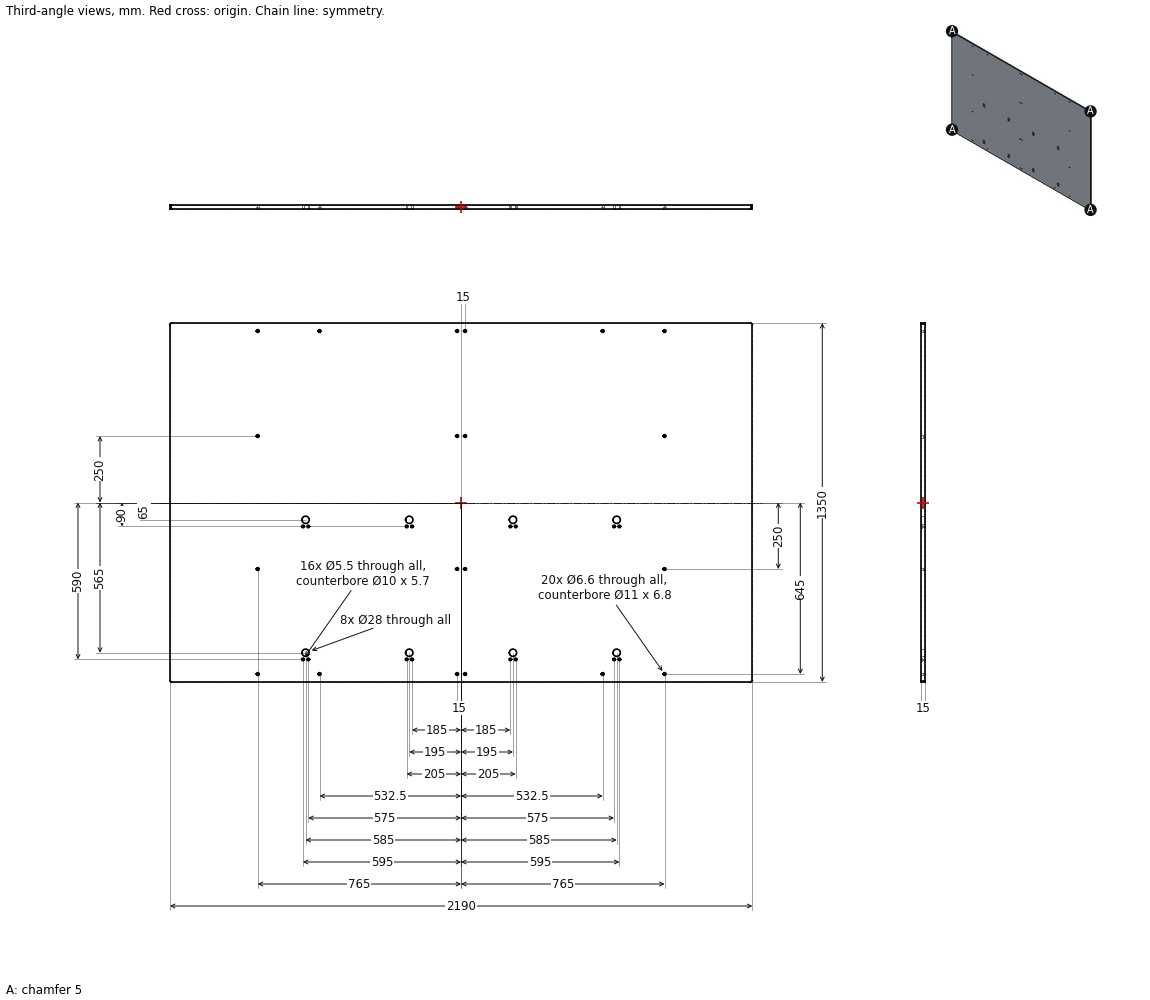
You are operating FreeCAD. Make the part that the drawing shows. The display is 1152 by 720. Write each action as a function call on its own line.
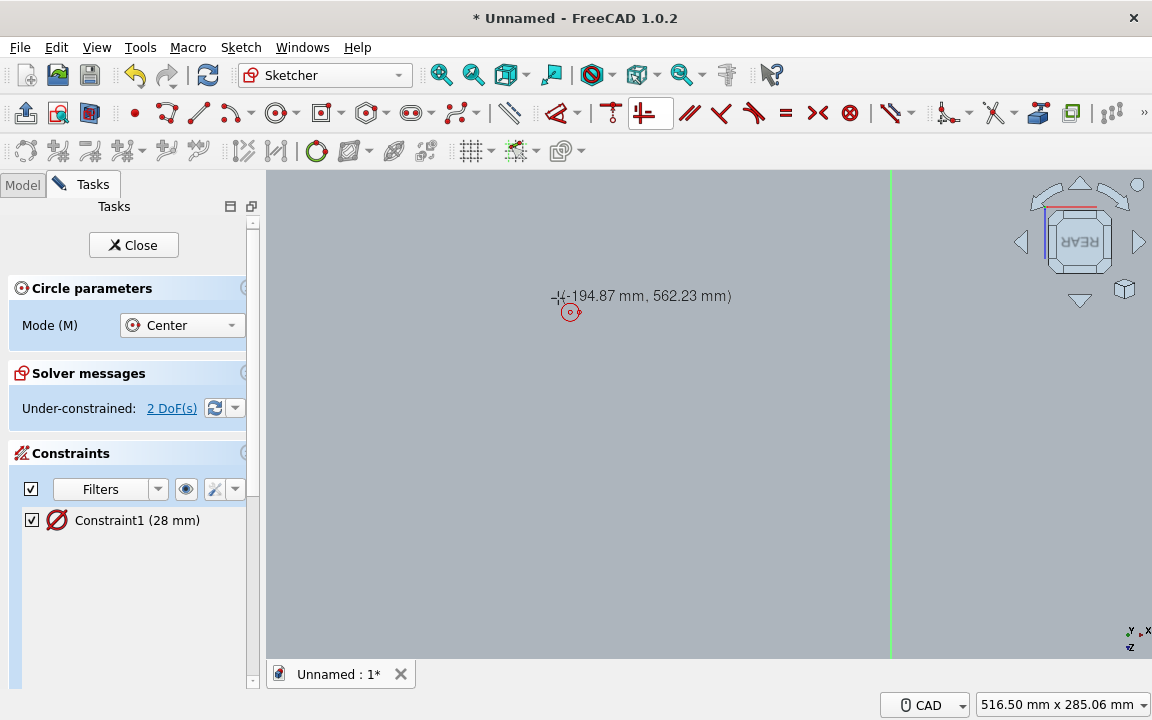
scroll(558, 298, down, 7)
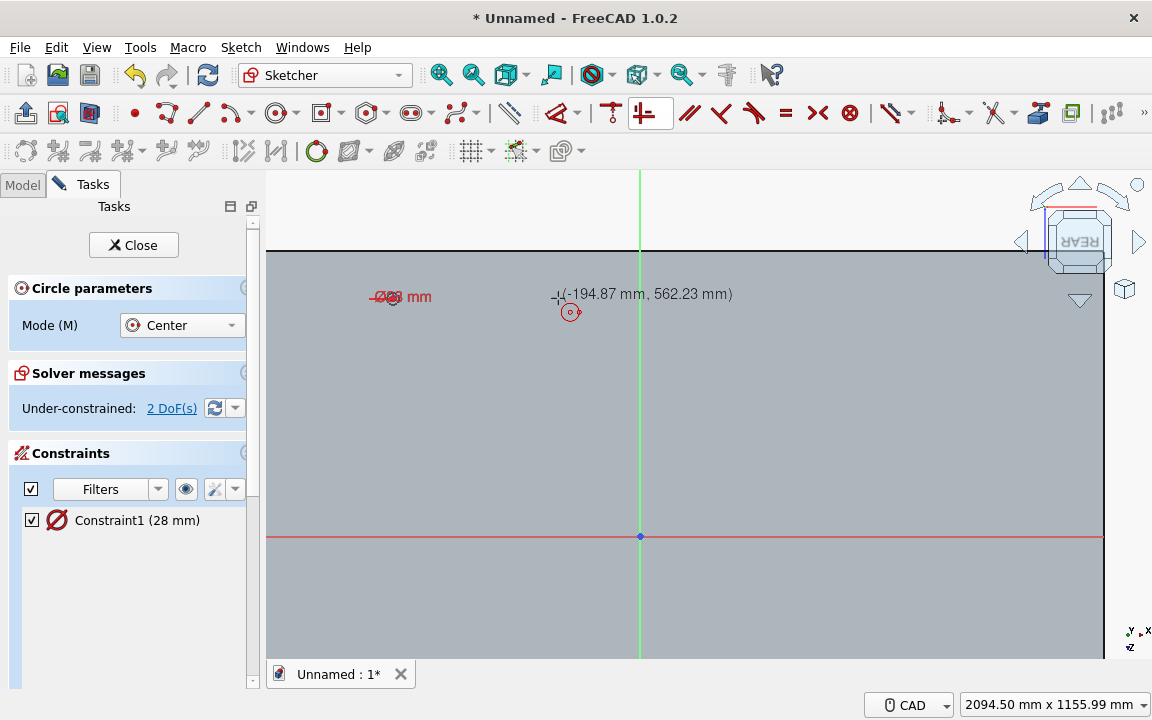
click(558, 298)
move(562, 294)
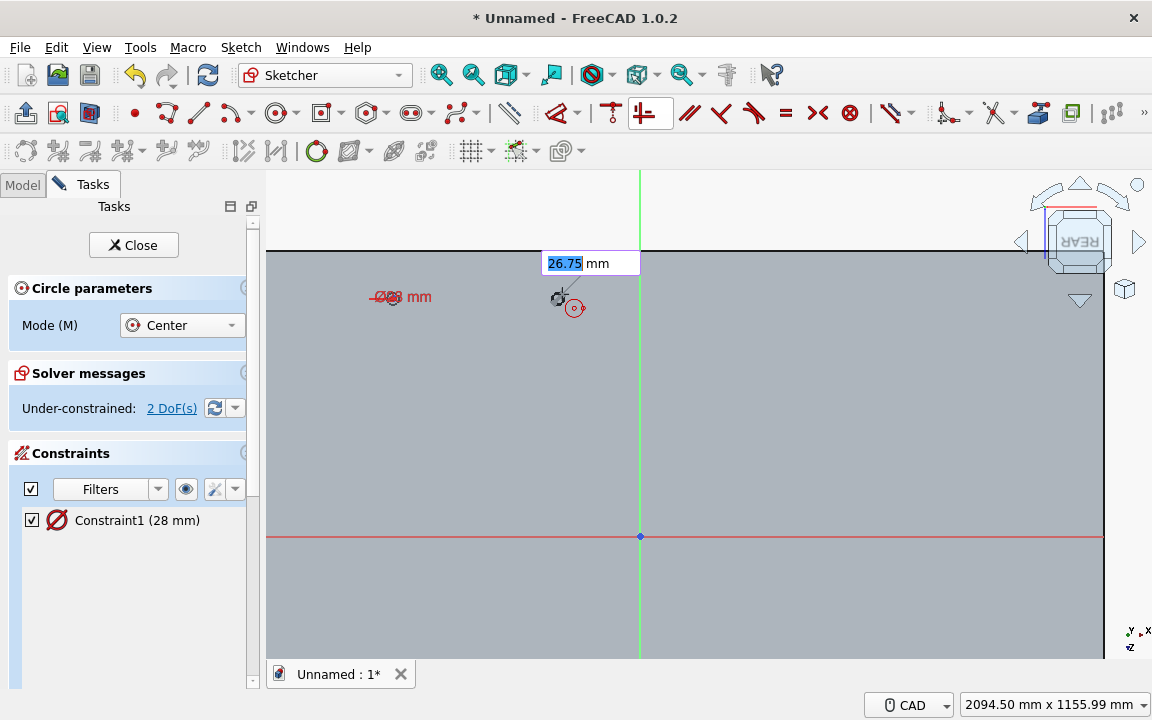
text(28)
key(Return)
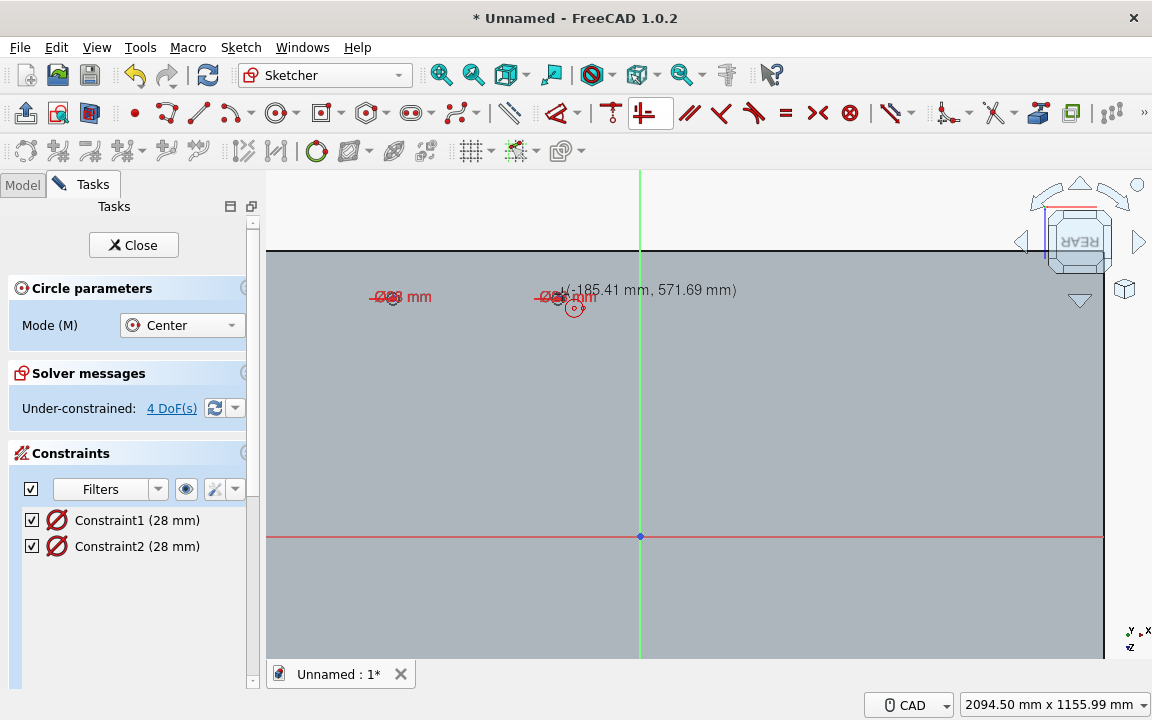
scroll(723, 298, up, 7)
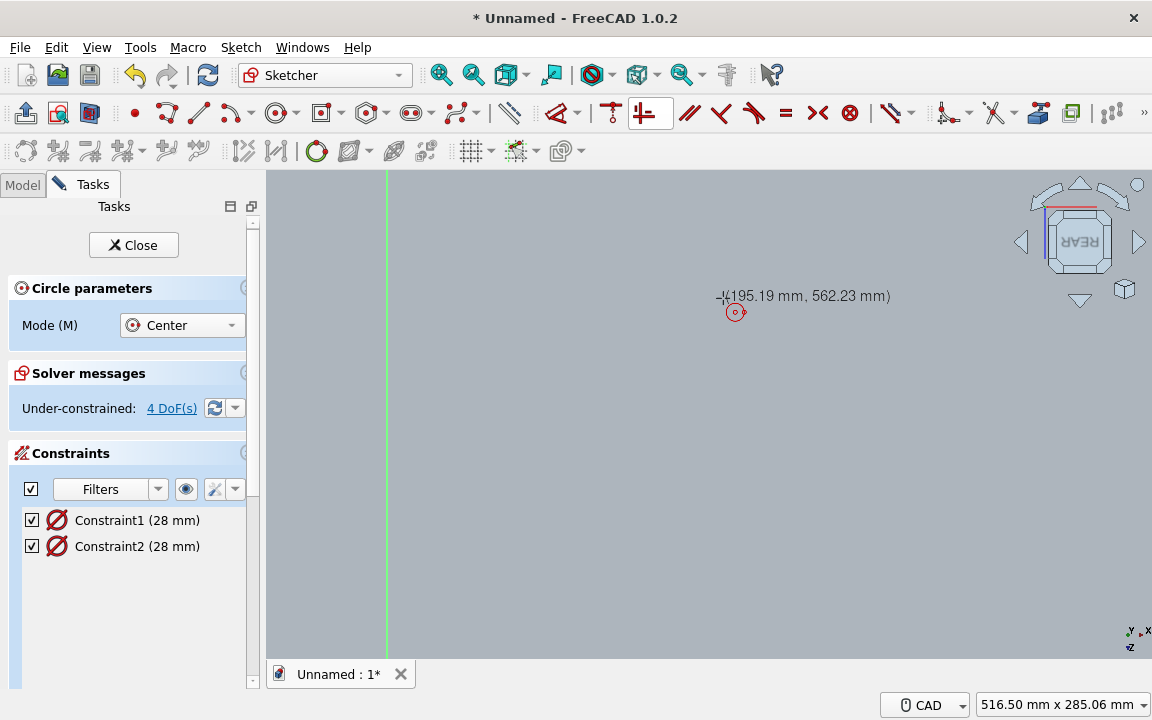
scroll(724, 298, down, 7)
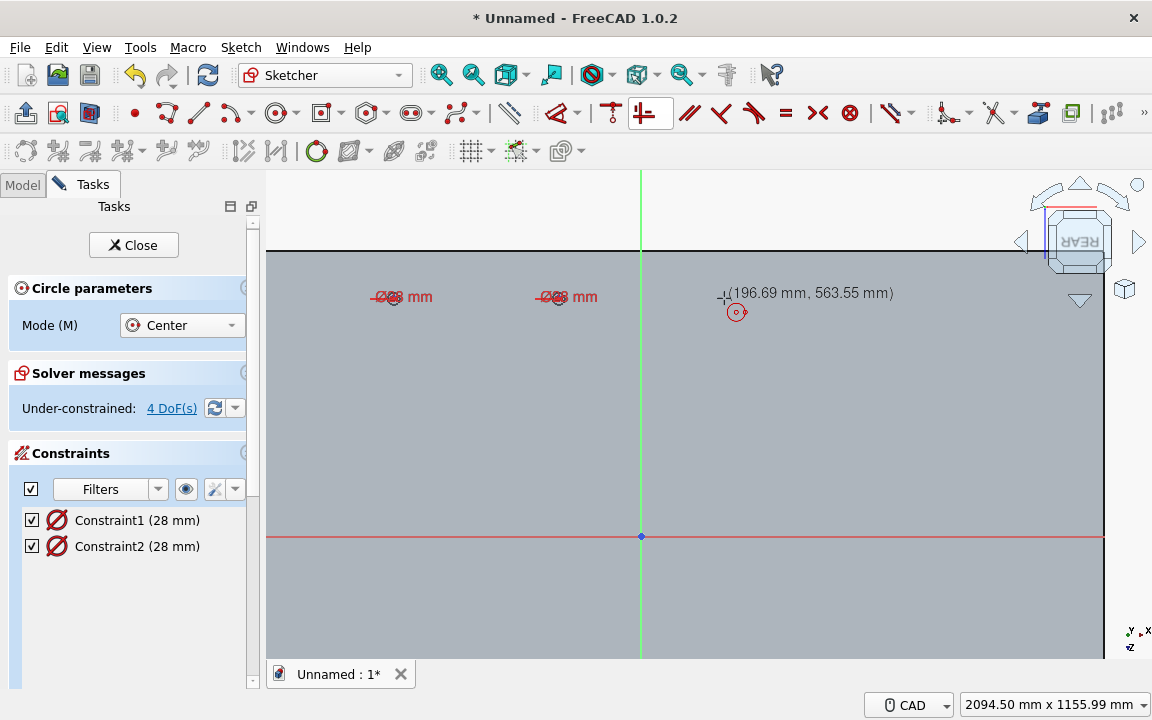
click(724, 298)
move(728, 294)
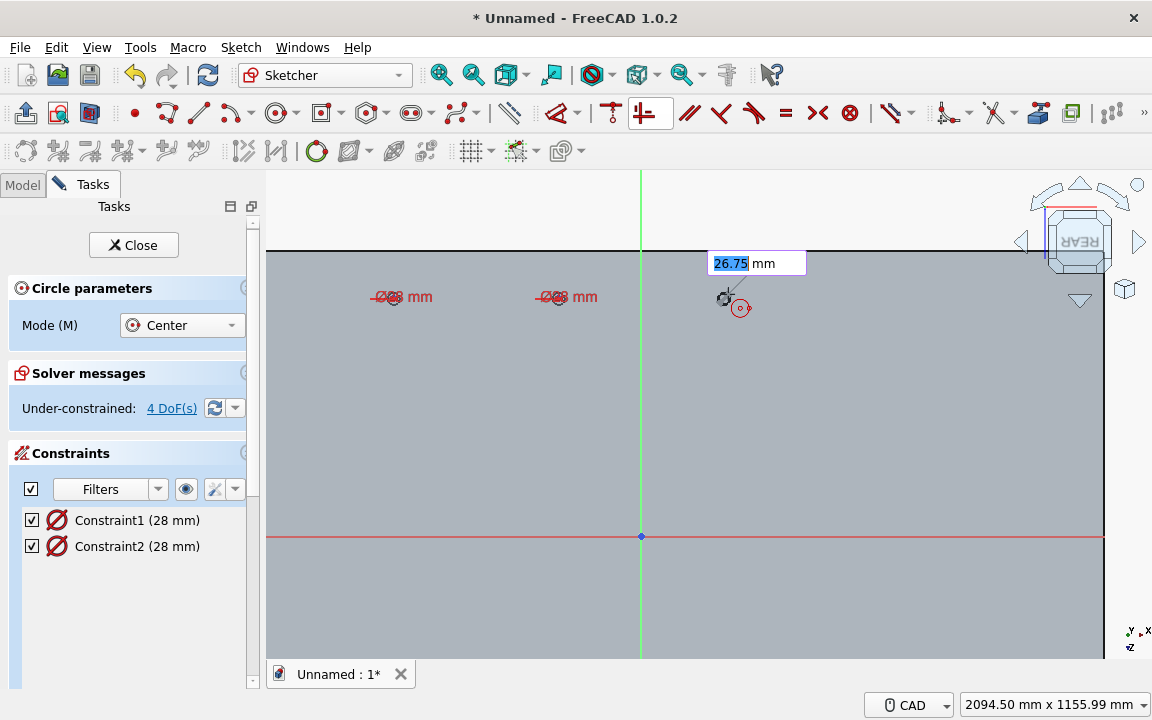
text(28)
key(Return)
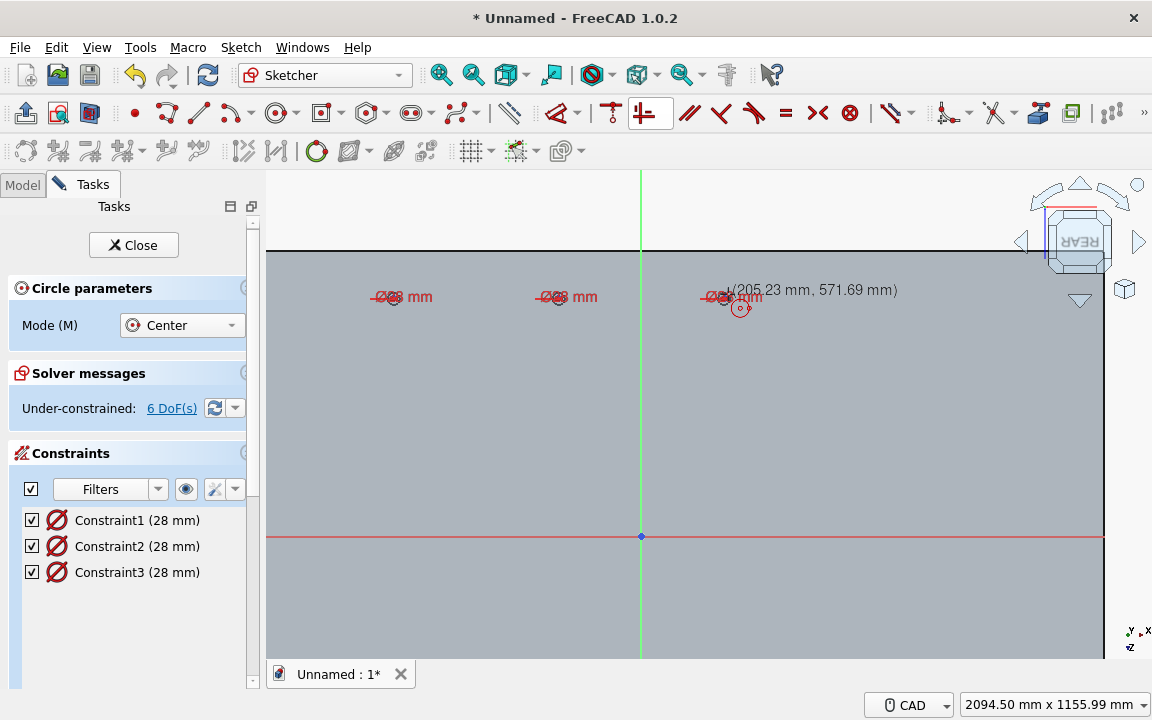
scroll(889, 298, up, 7)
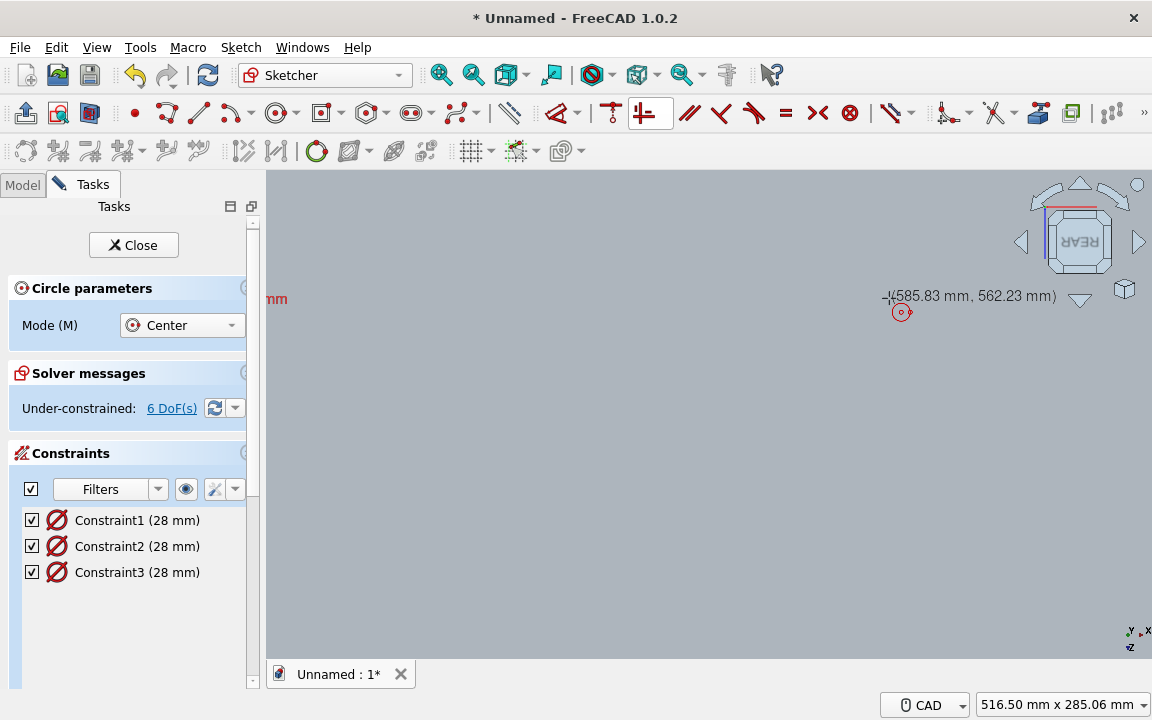
scroll(889, 298, down, 7)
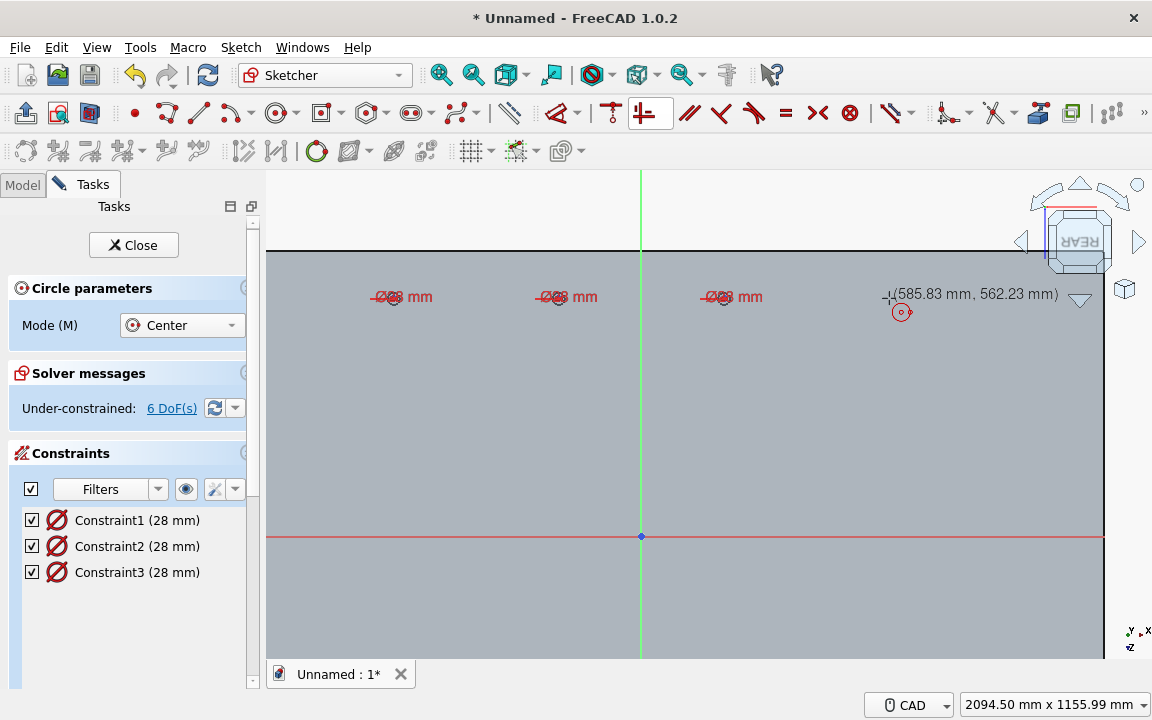
click(889, 298)
move(893, 294)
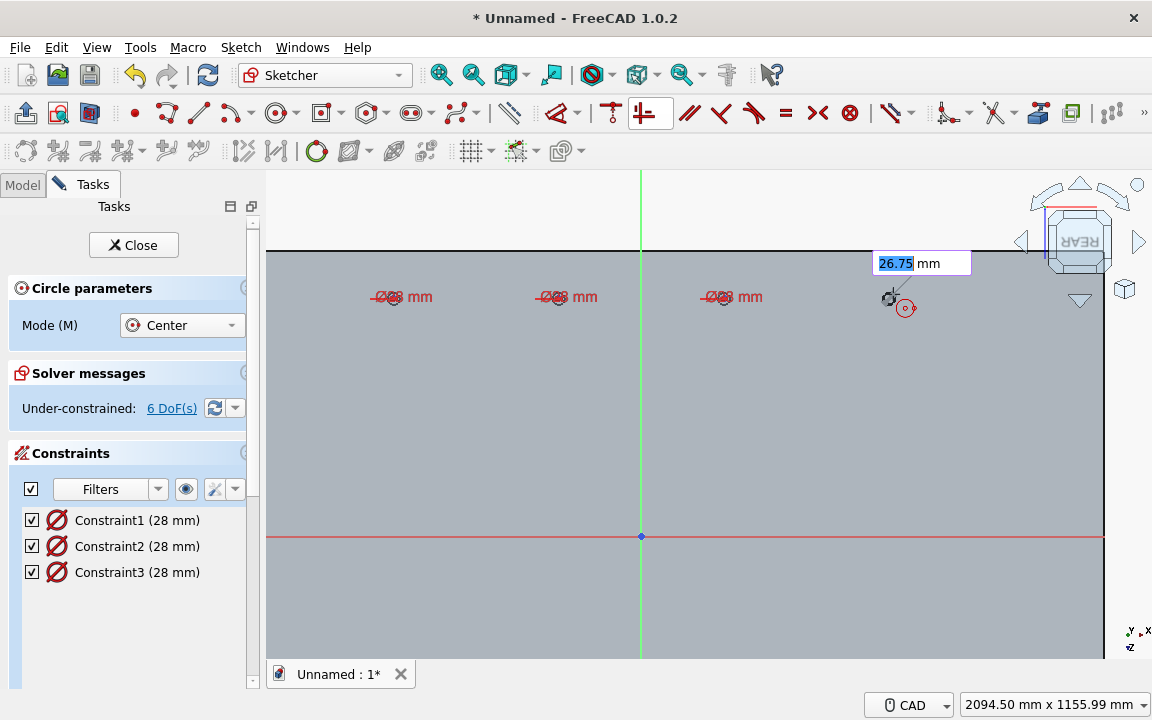
text(28)
key(Return)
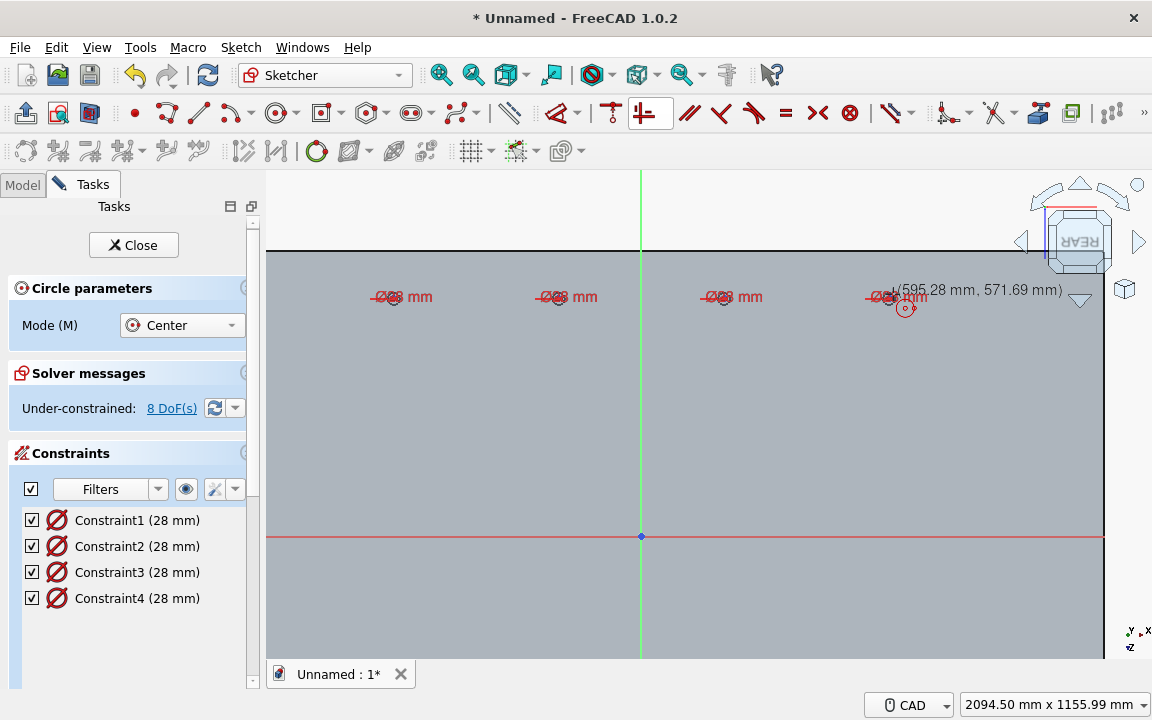
scroll(394, 509, up, 7)